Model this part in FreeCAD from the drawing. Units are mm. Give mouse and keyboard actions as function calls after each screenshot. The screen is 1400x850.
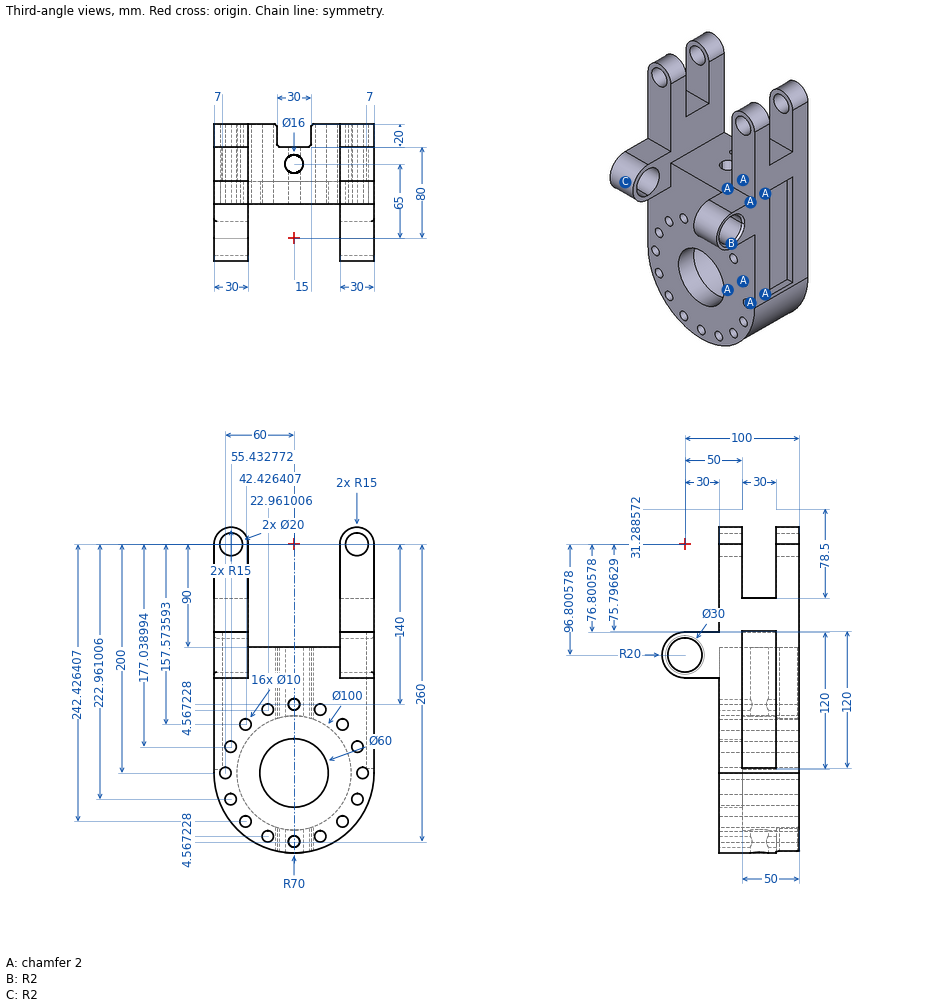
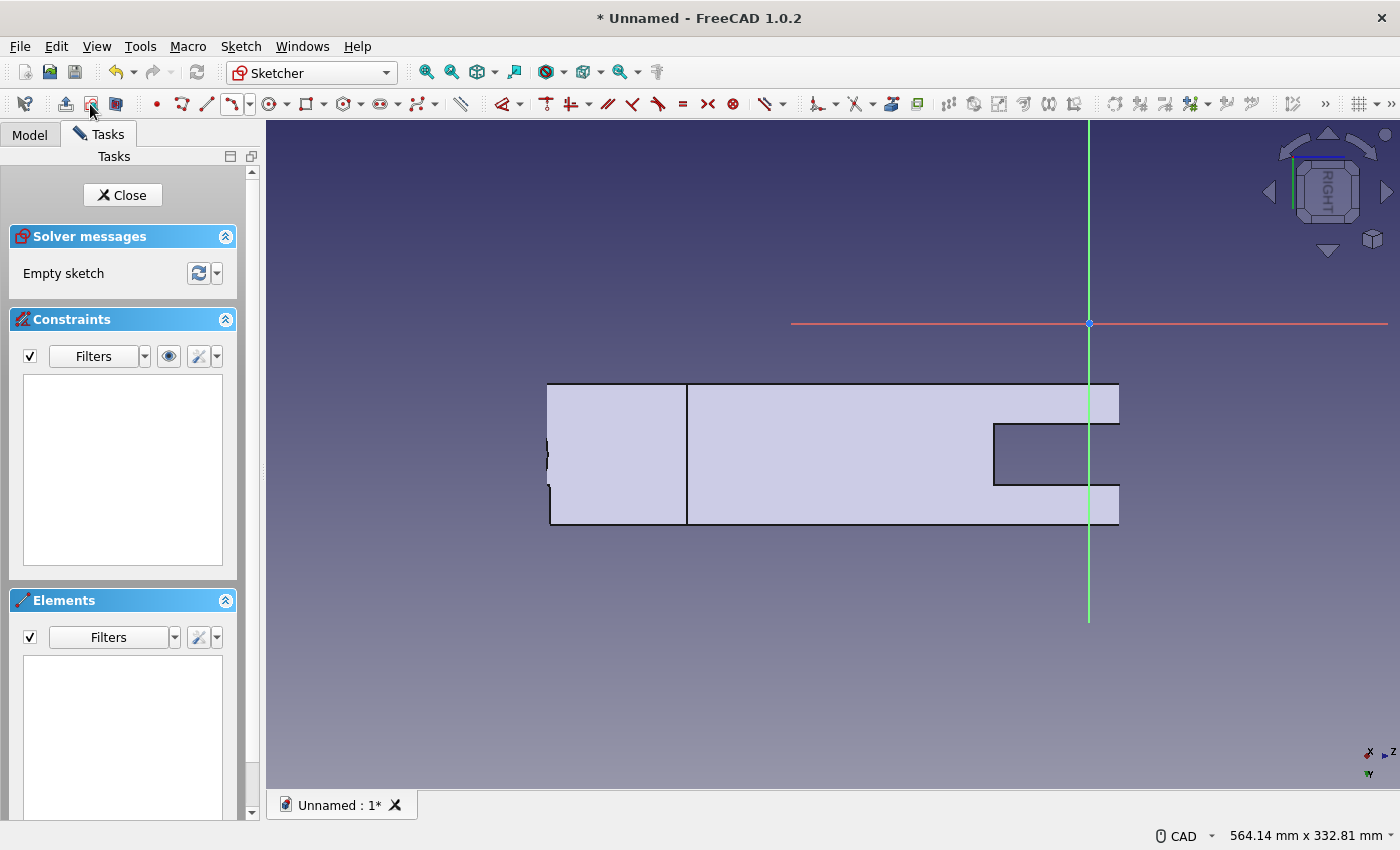
scroll(1048, 343, up, 3)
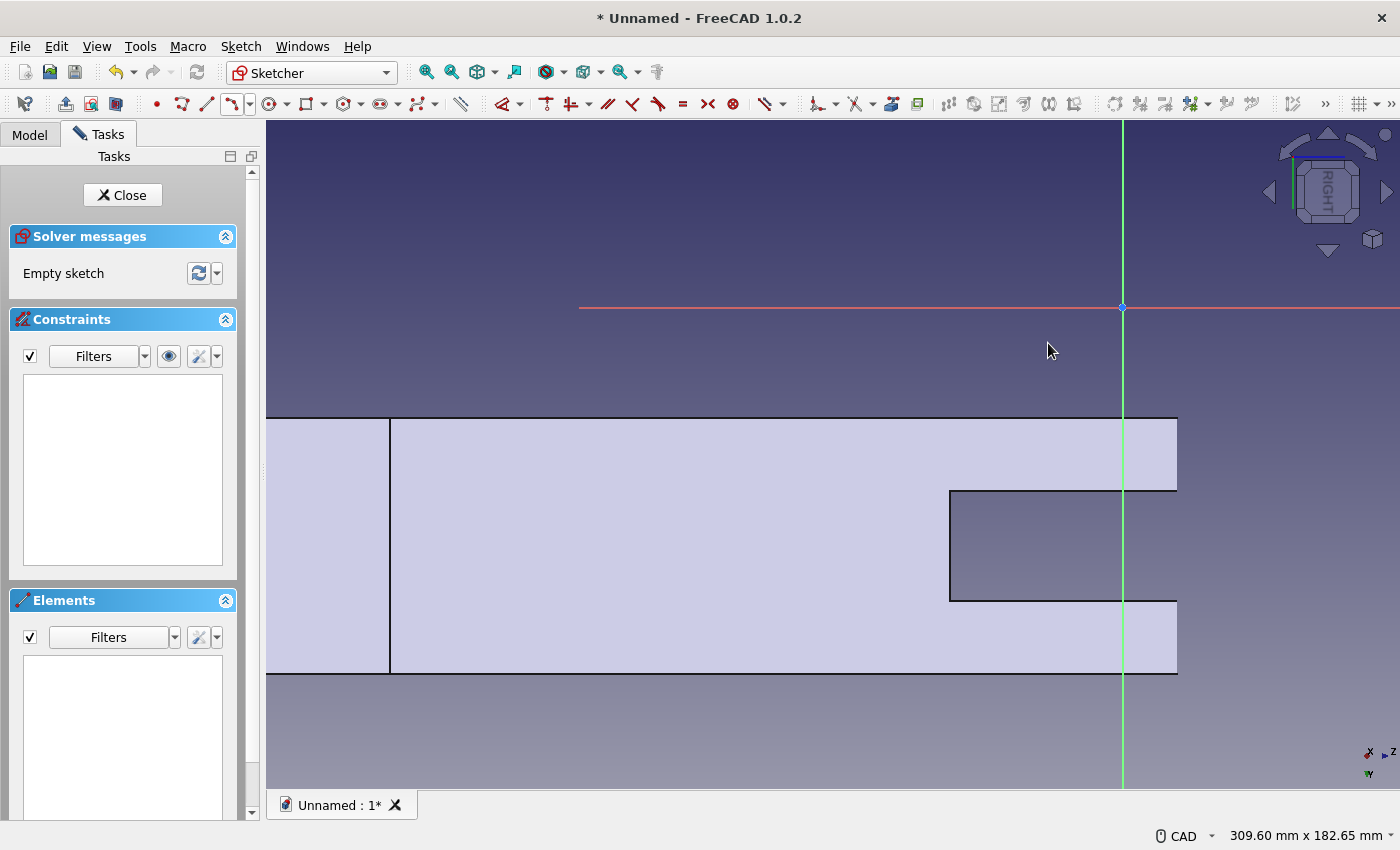
key(g)
key(r)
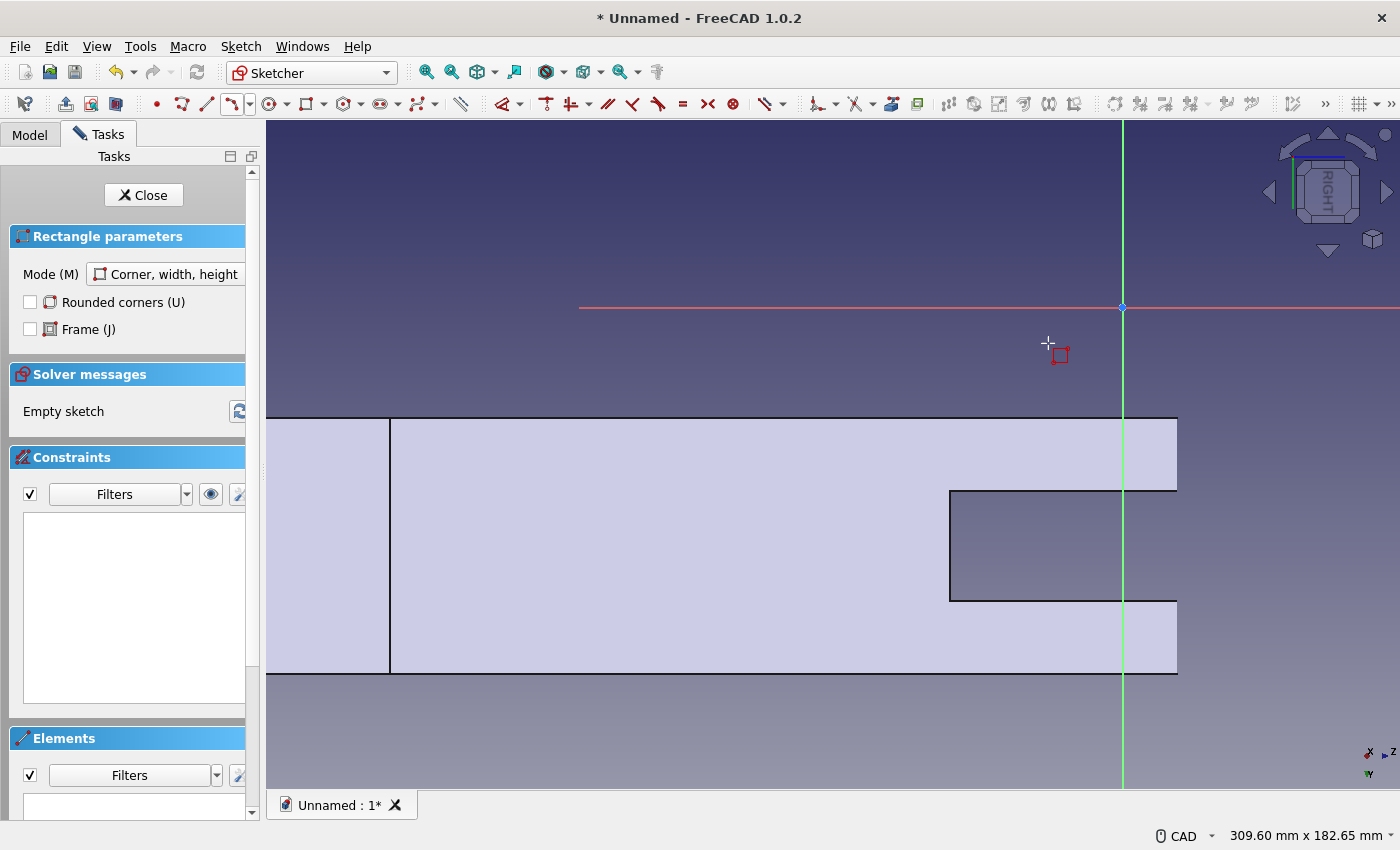
click(406, 491)
click(845, 601)
key(Escape)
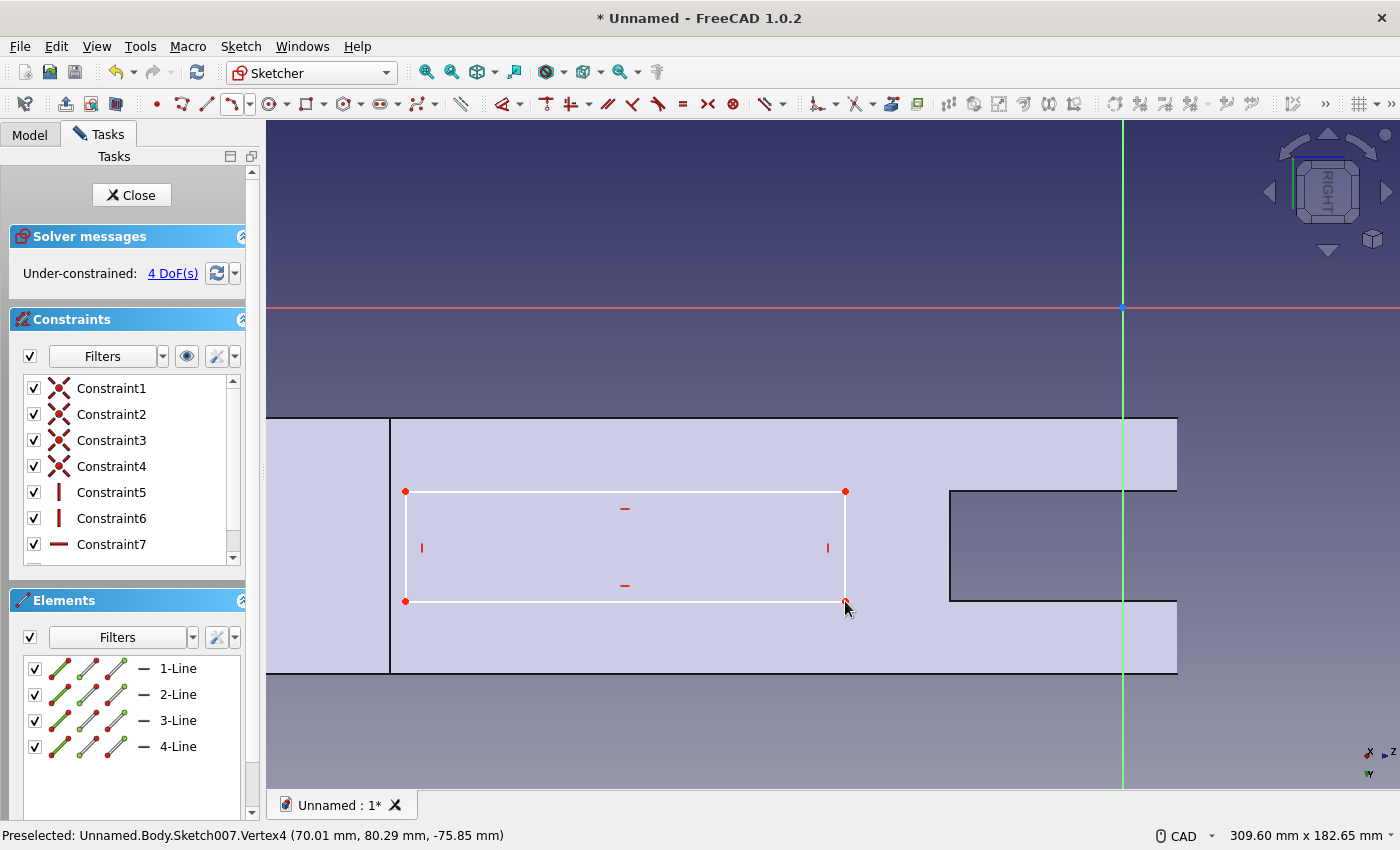
key(d)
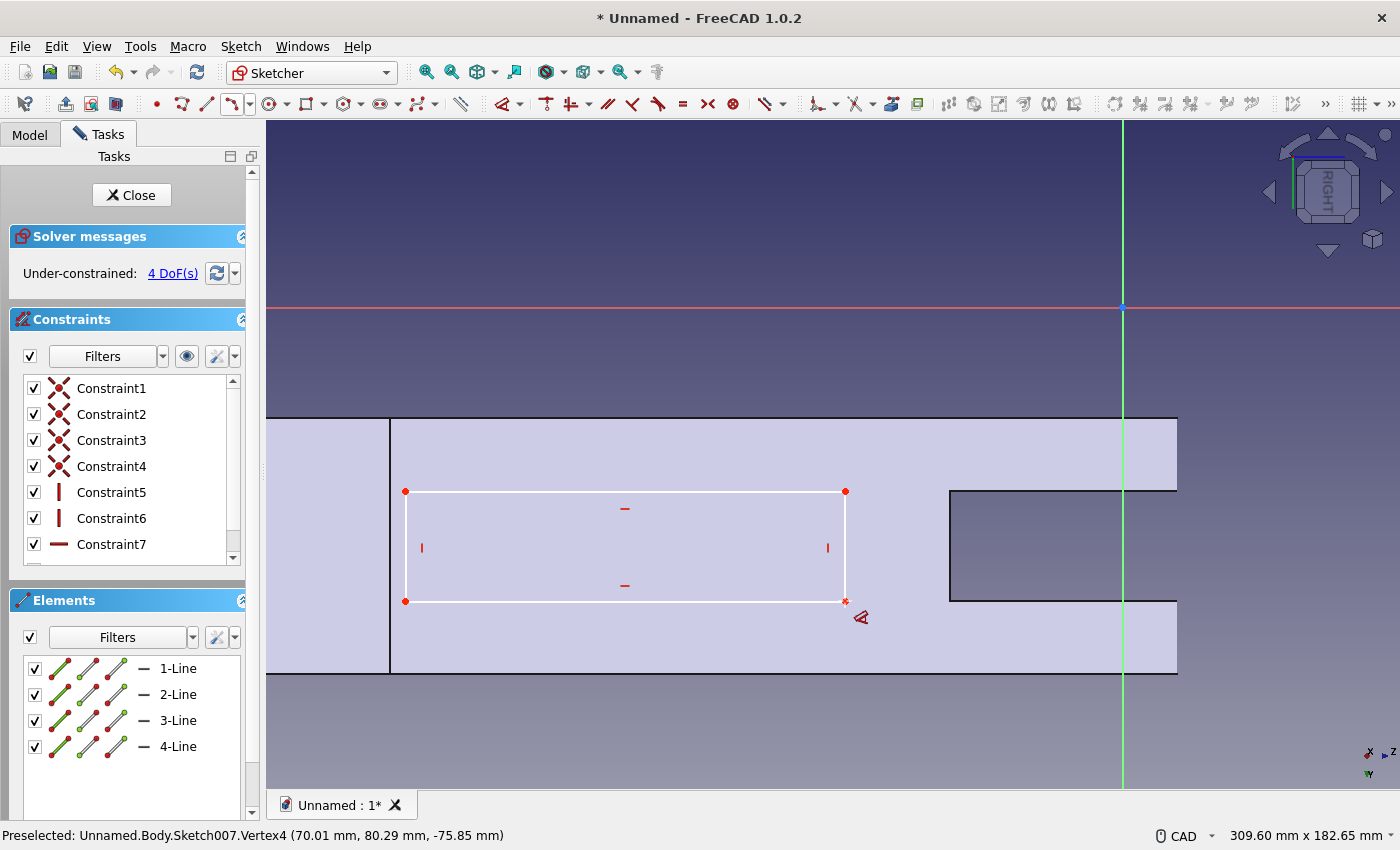
click(406, 525)
click(372, 547)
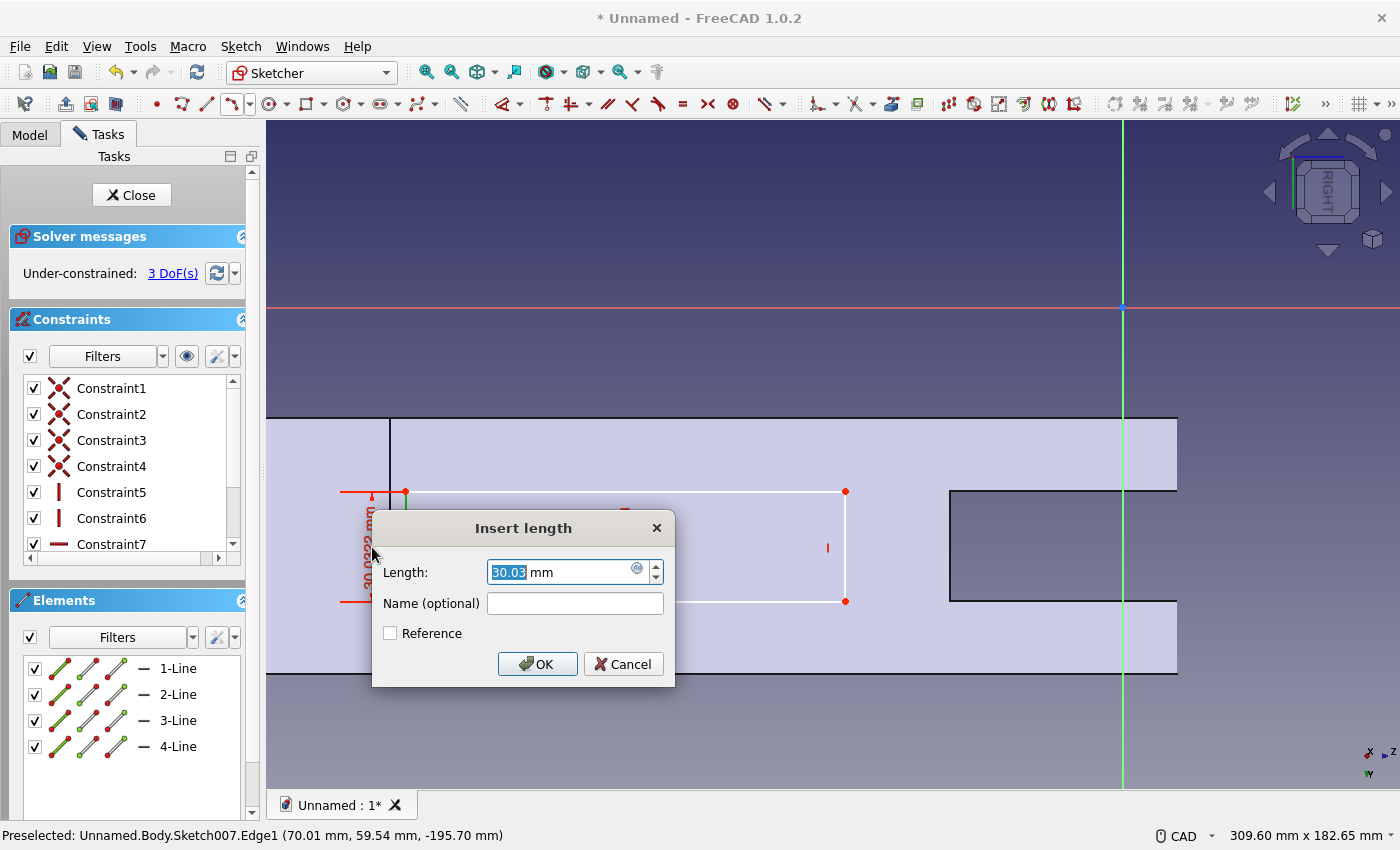
text(30)
key(Return)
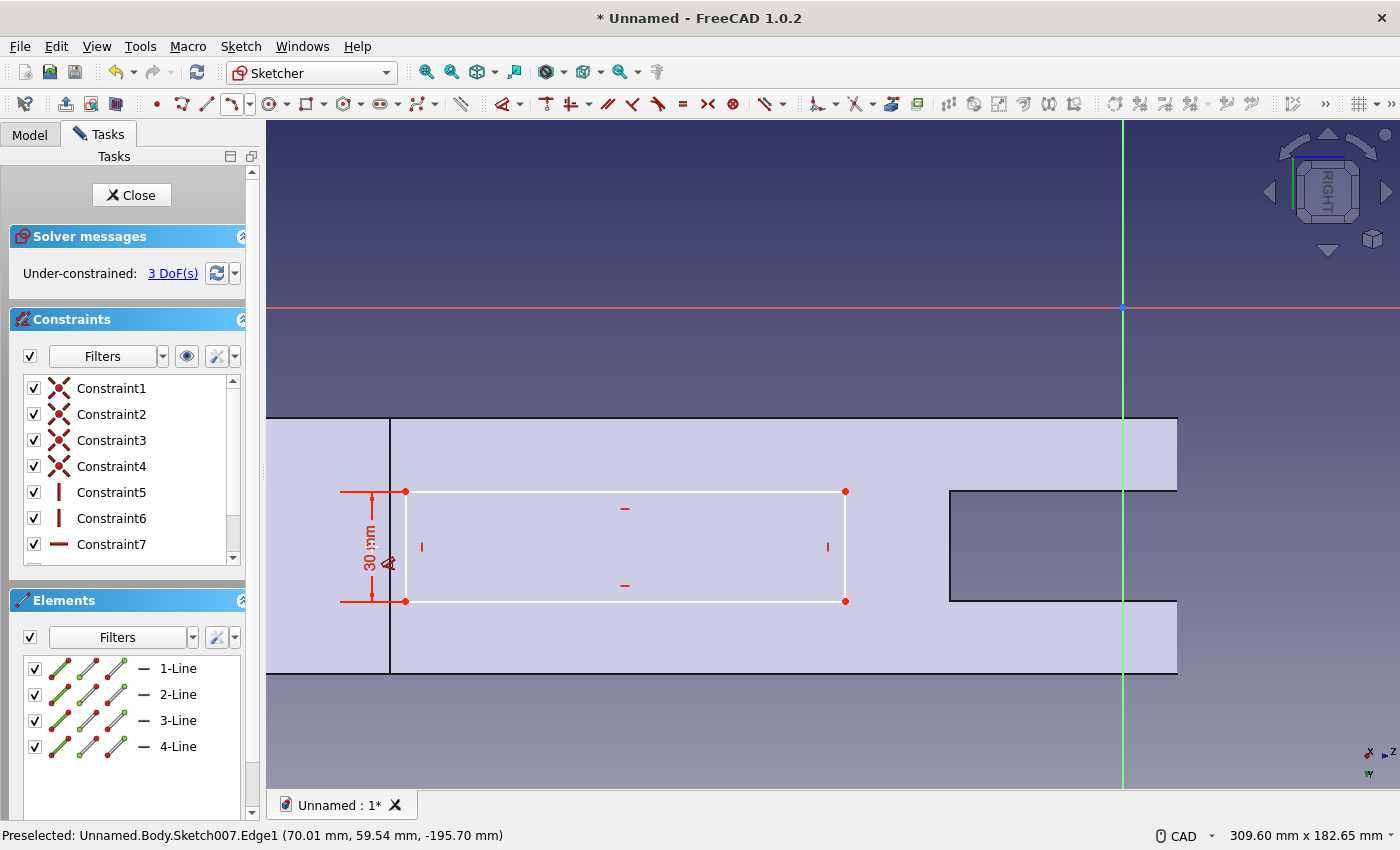
click(538, 602)
click(625, 636)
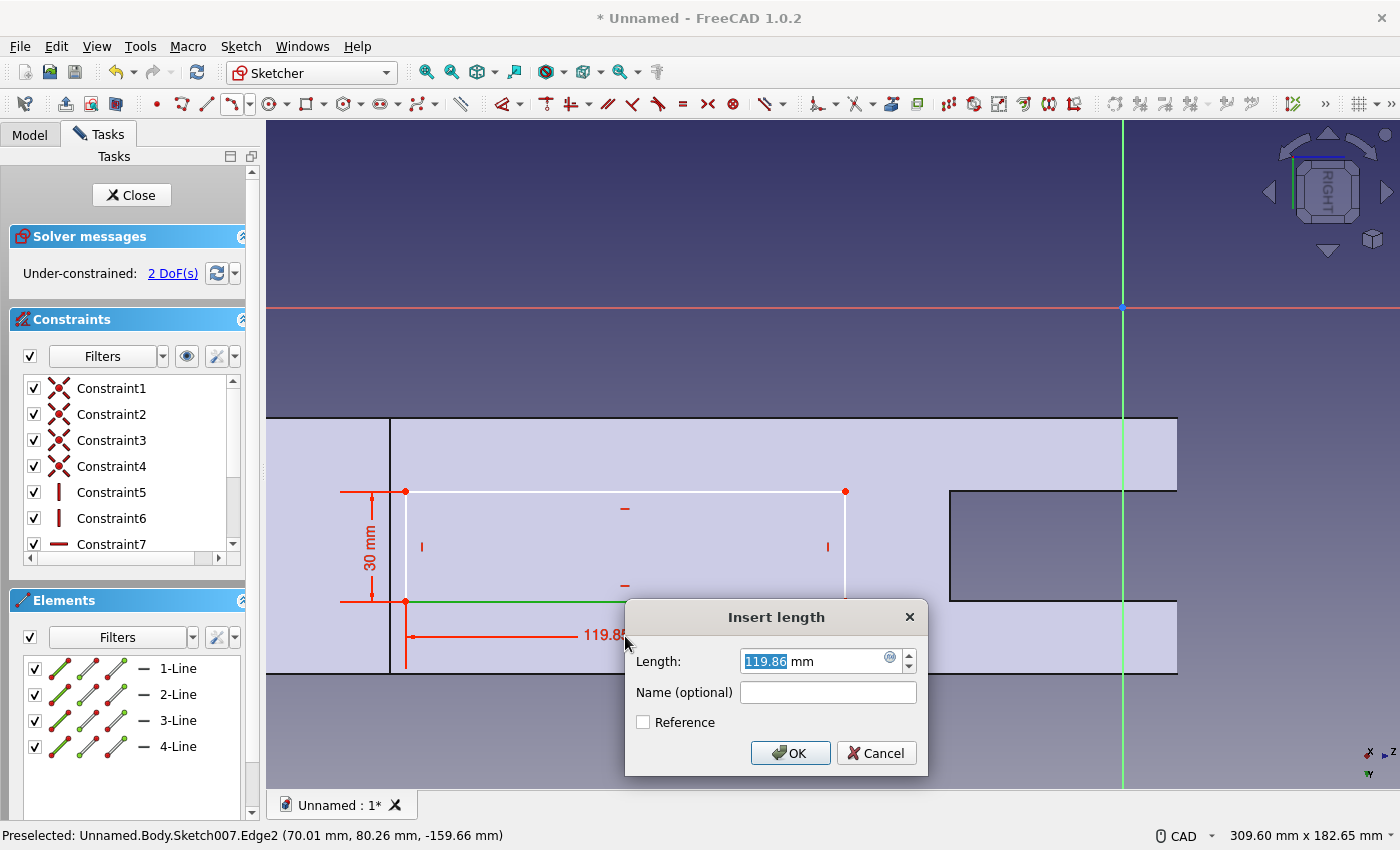
text(120)
key(Return)